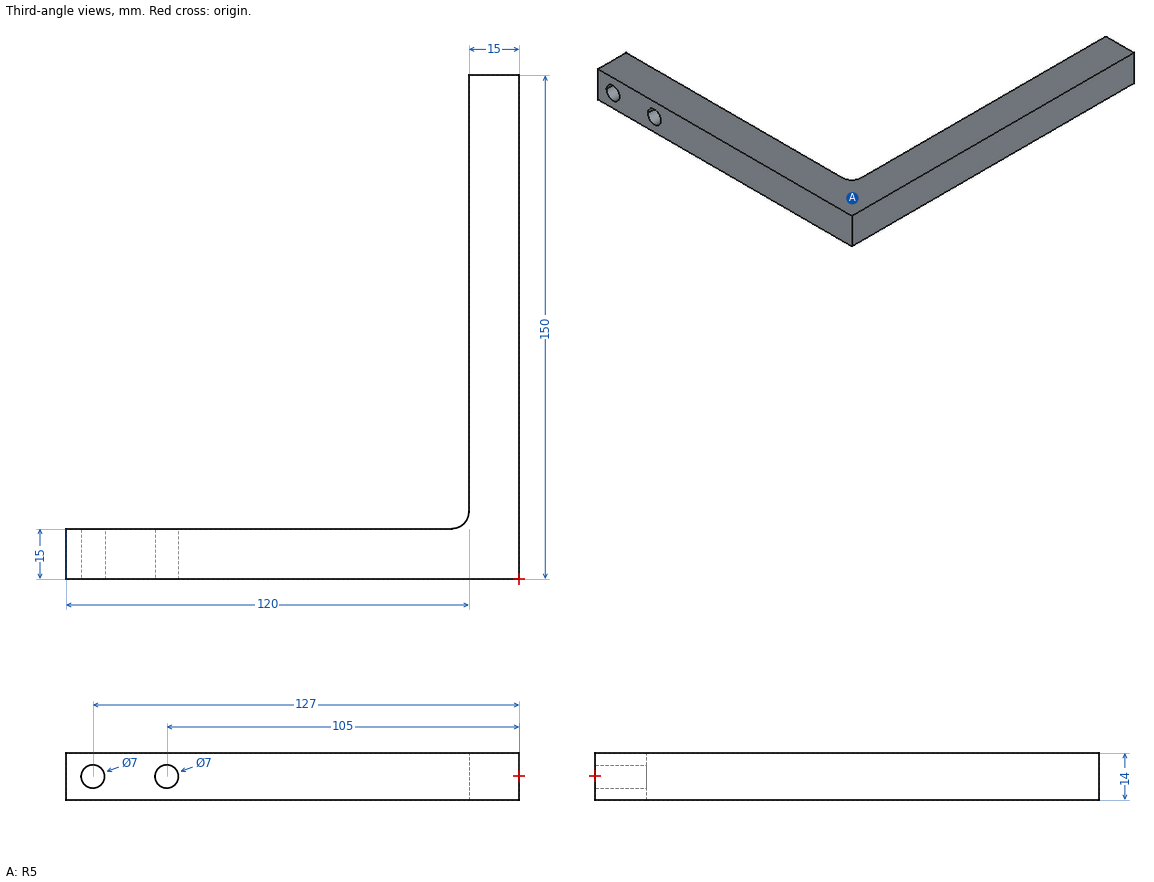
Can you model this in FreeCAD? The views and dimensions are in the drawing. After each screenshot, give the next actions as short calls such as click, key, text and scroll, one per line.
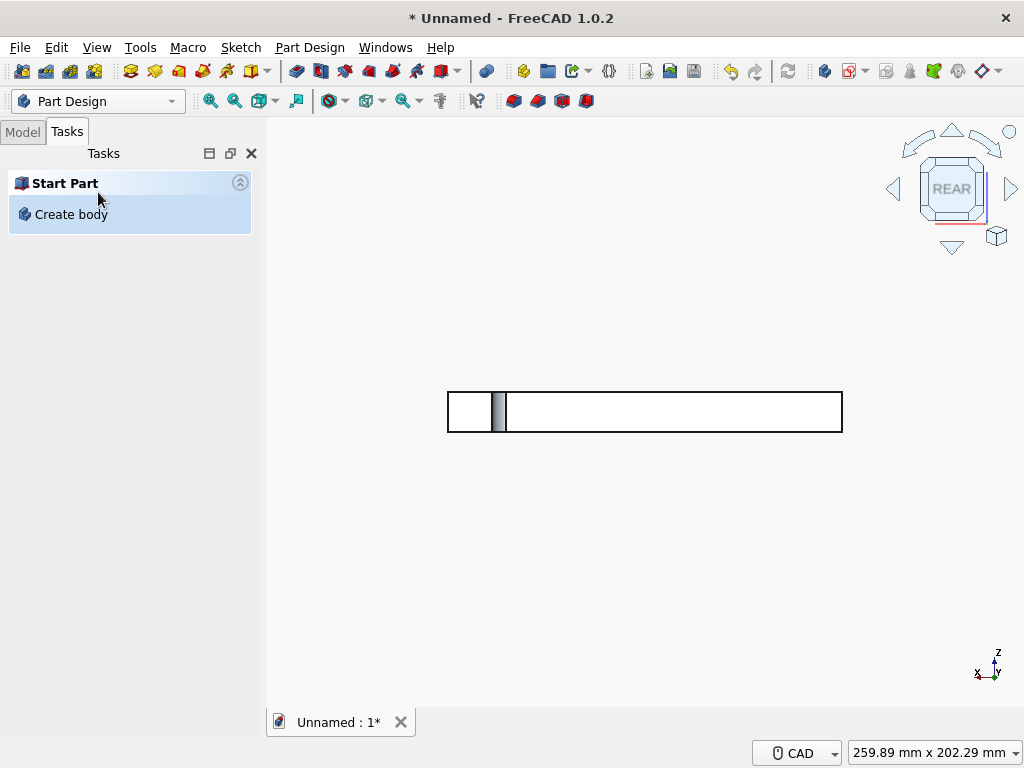
click(530, 411)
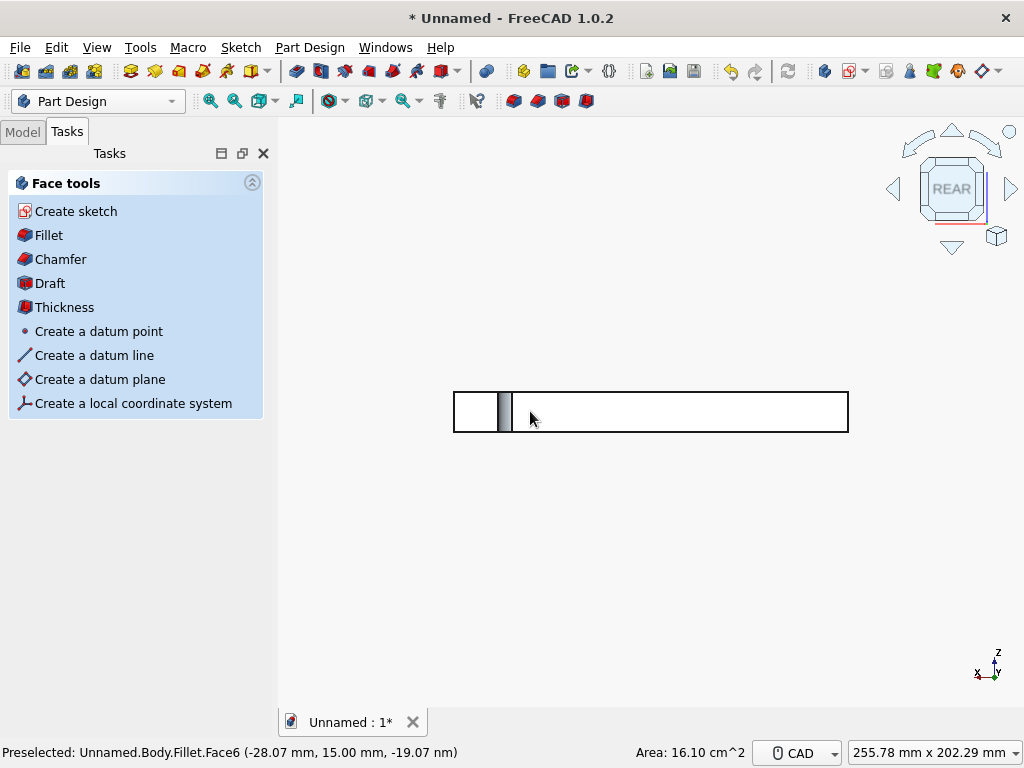
click(850, 72)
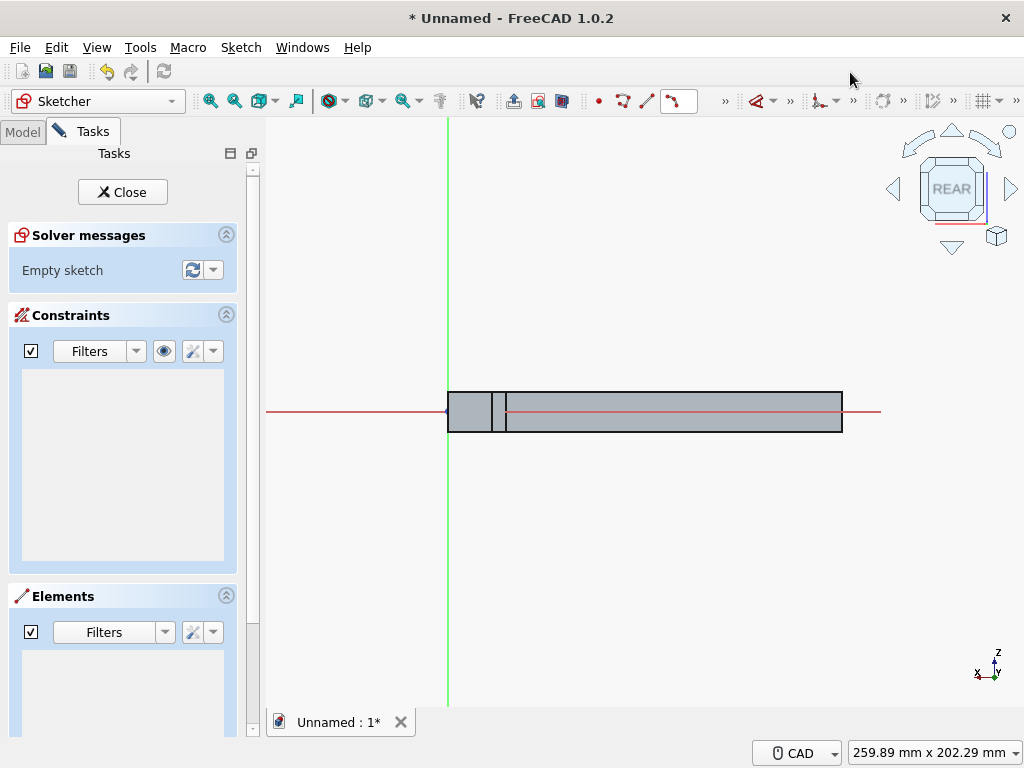
scroll(831, 412, up, 15)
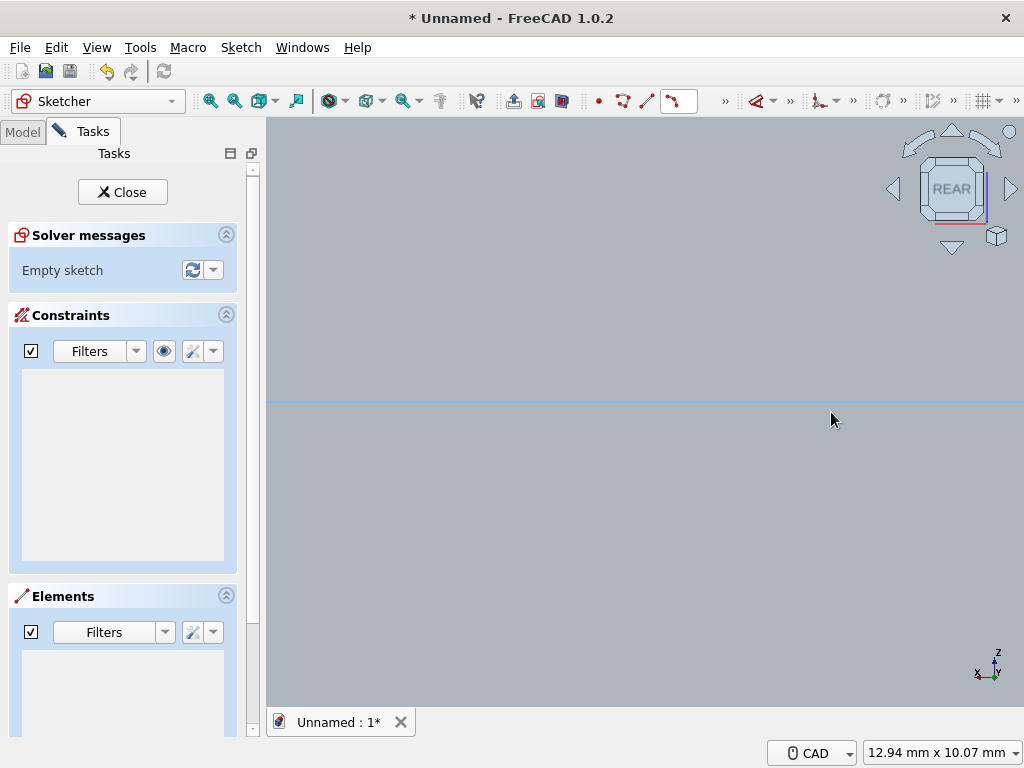
key(g)
key(c)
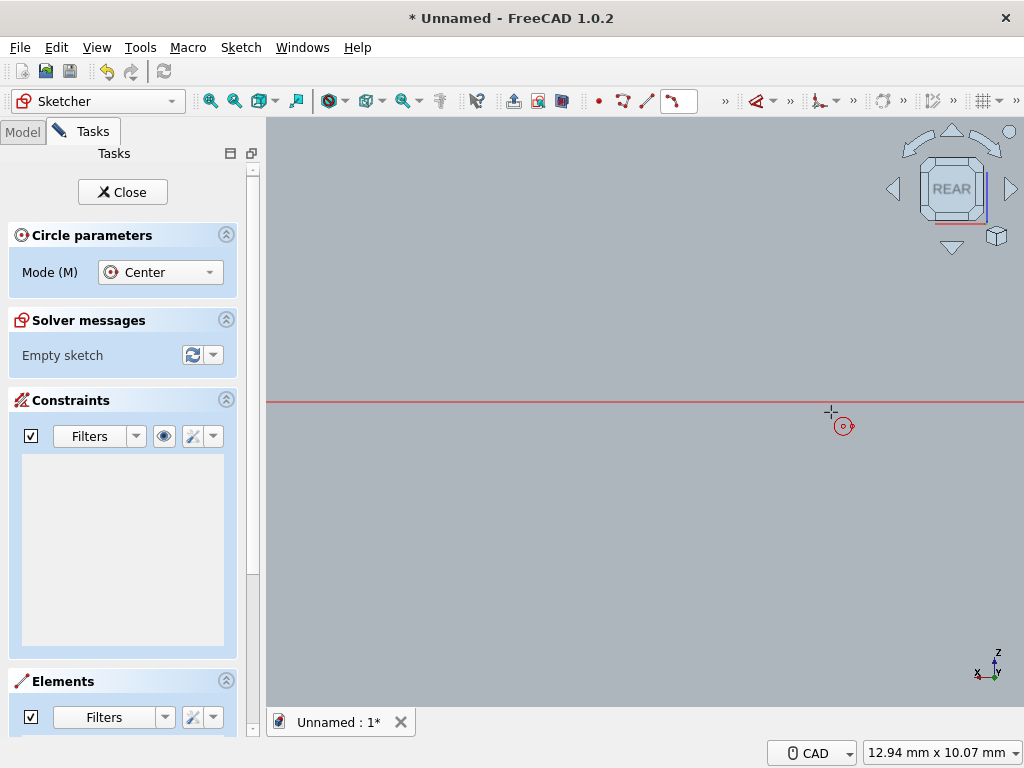
click(566, 402)
click(711, 257)
key(Escape)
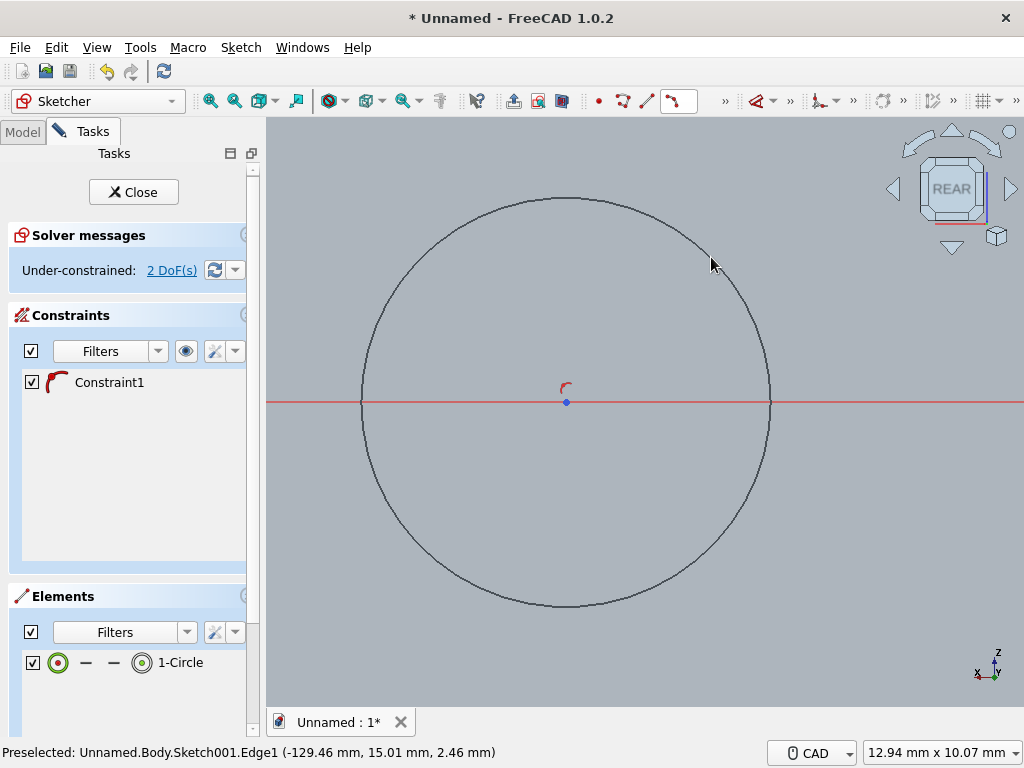
click(756, 102)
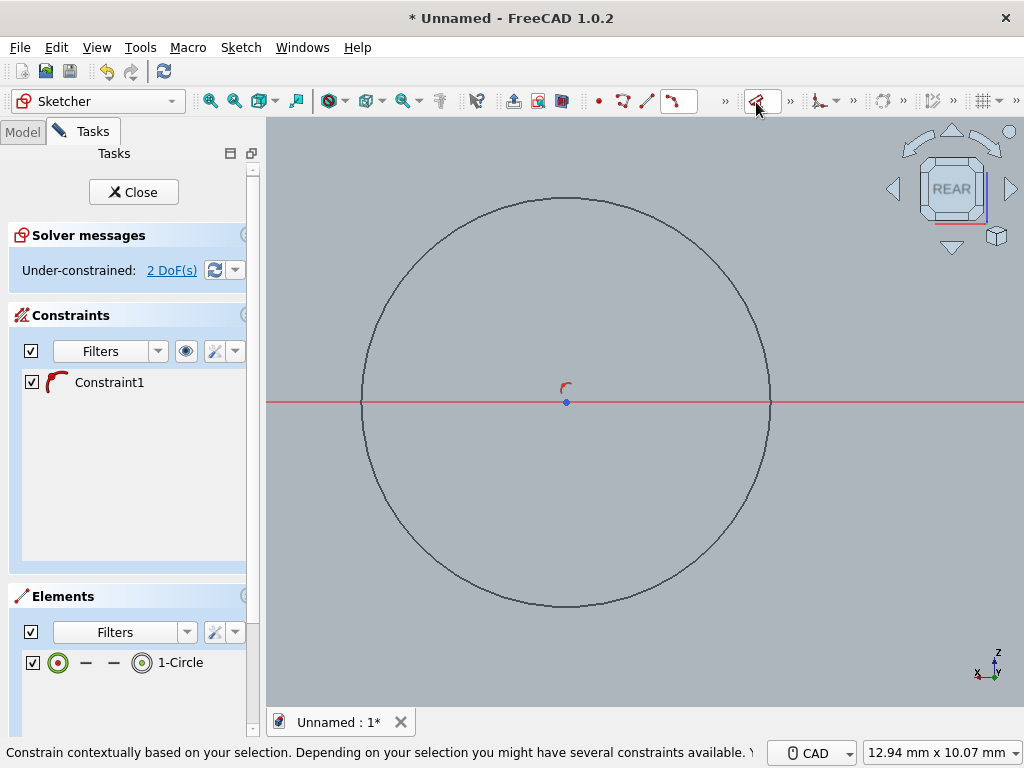
click(710, 257)
click(733, 234)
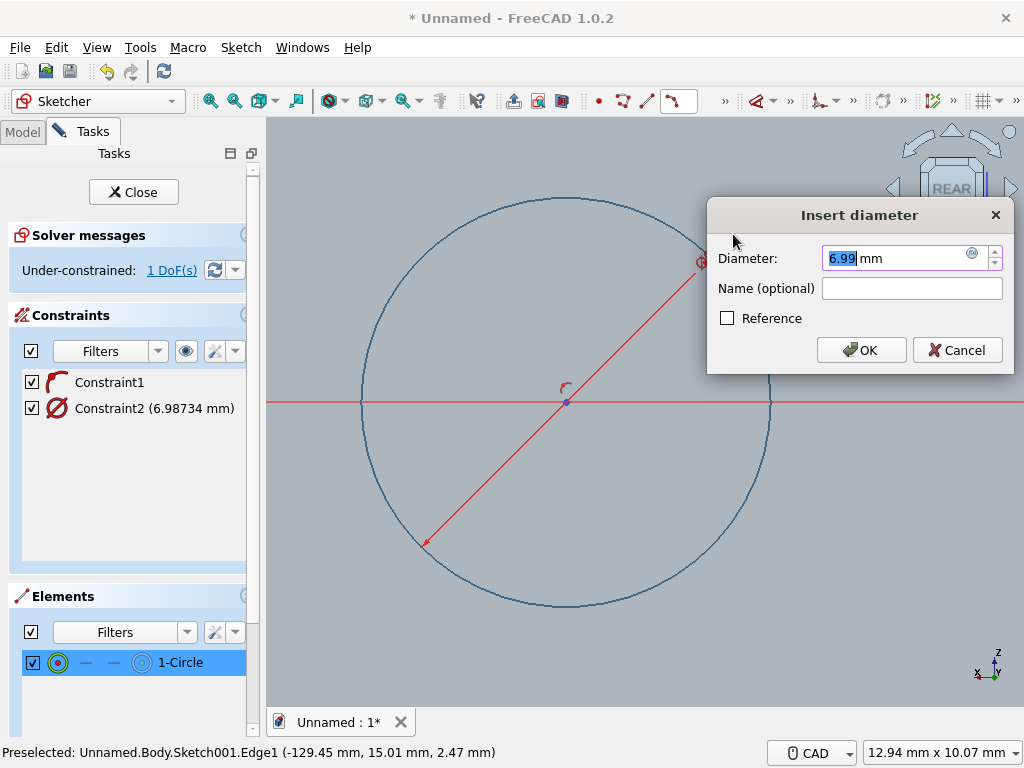
text(7)
key(Return)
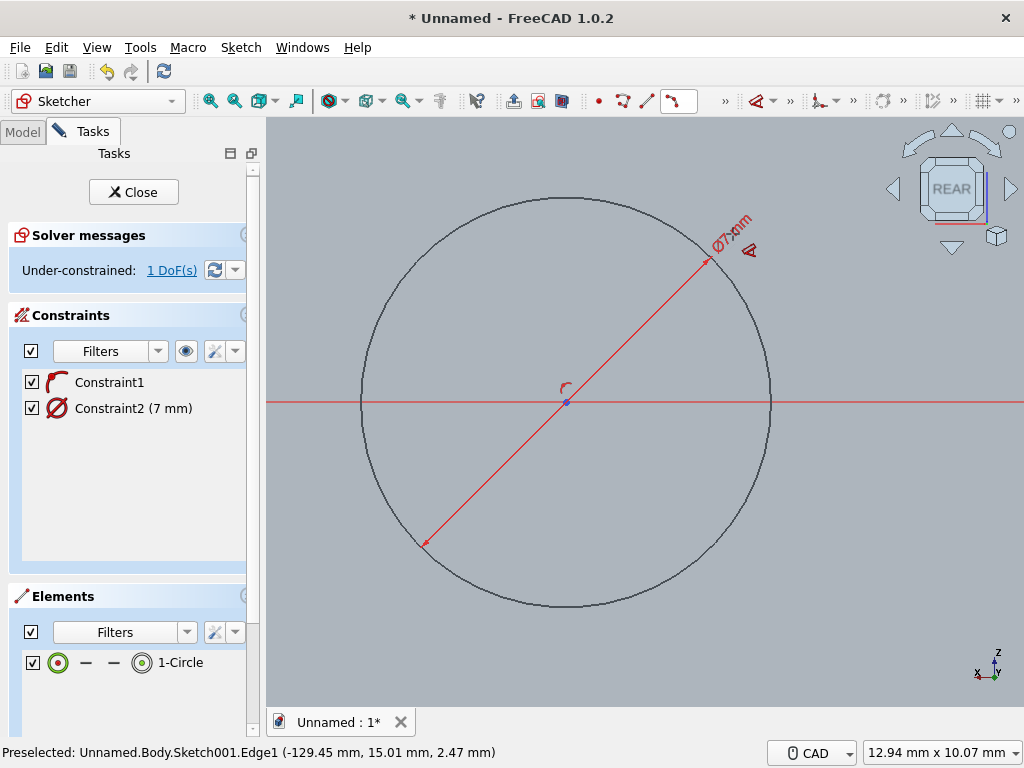
click(566, 402)
click(430, 436)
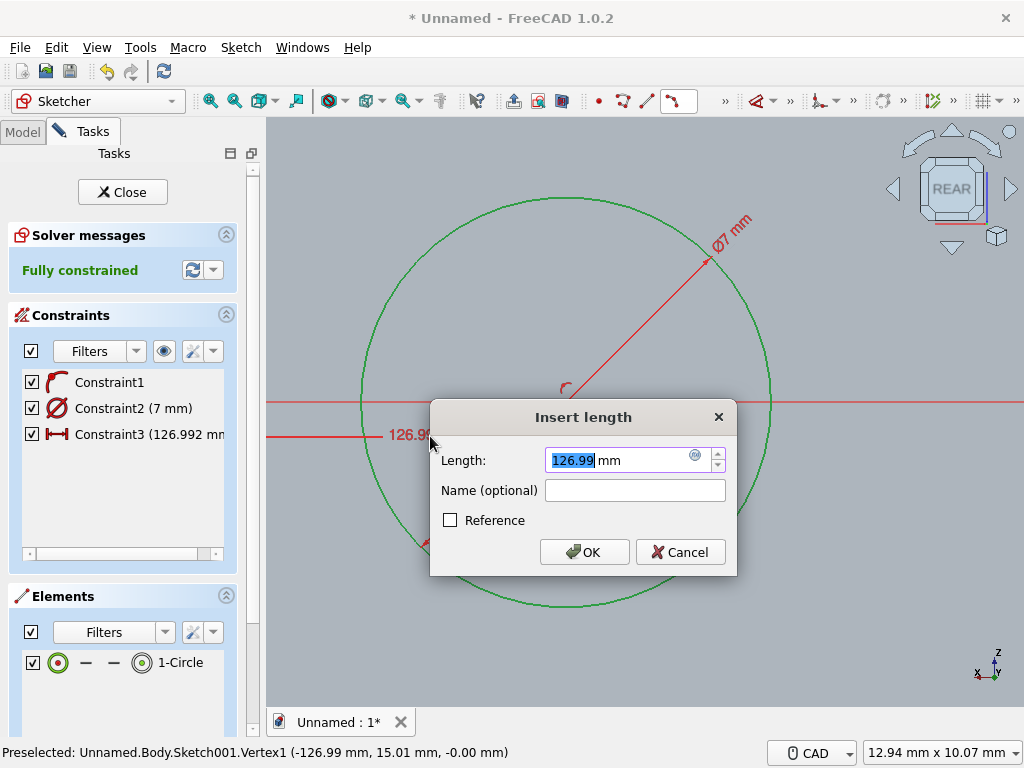
text(127)
key(Return)
key(Escape)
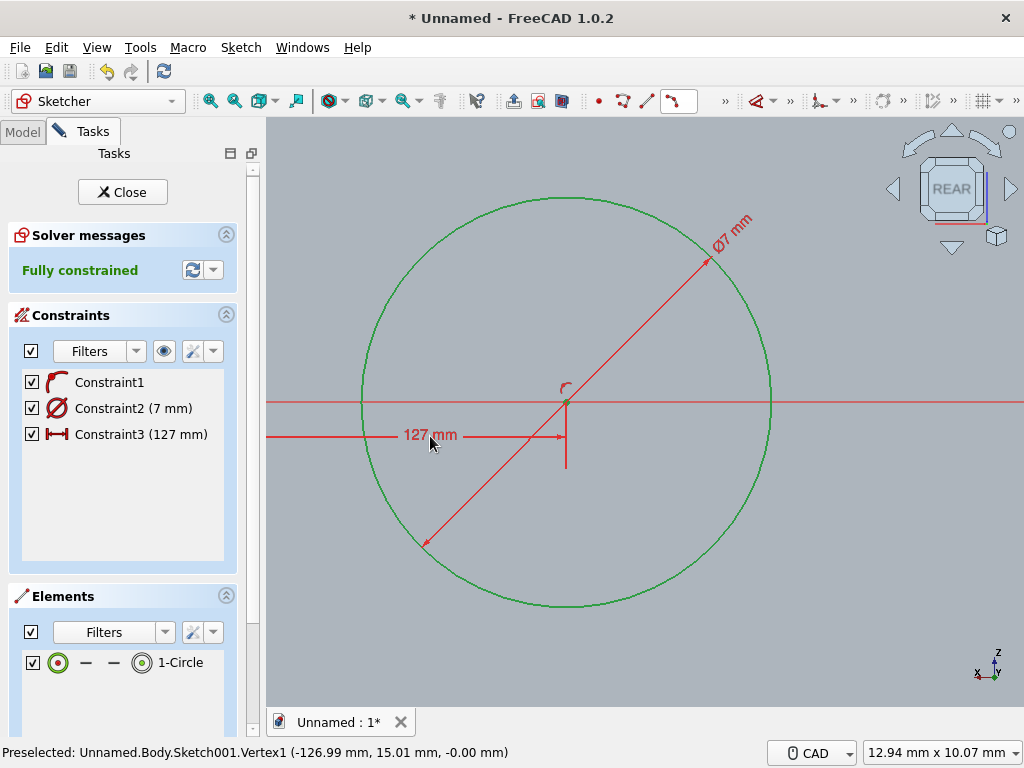
click(123, 192)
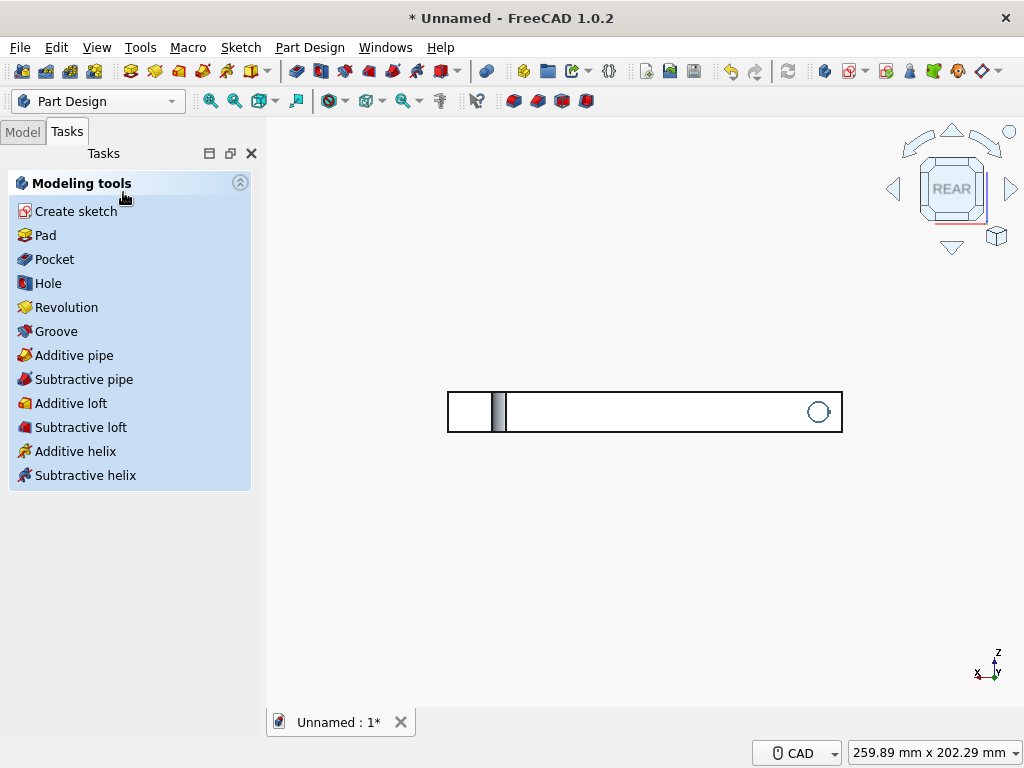
click(298, 72)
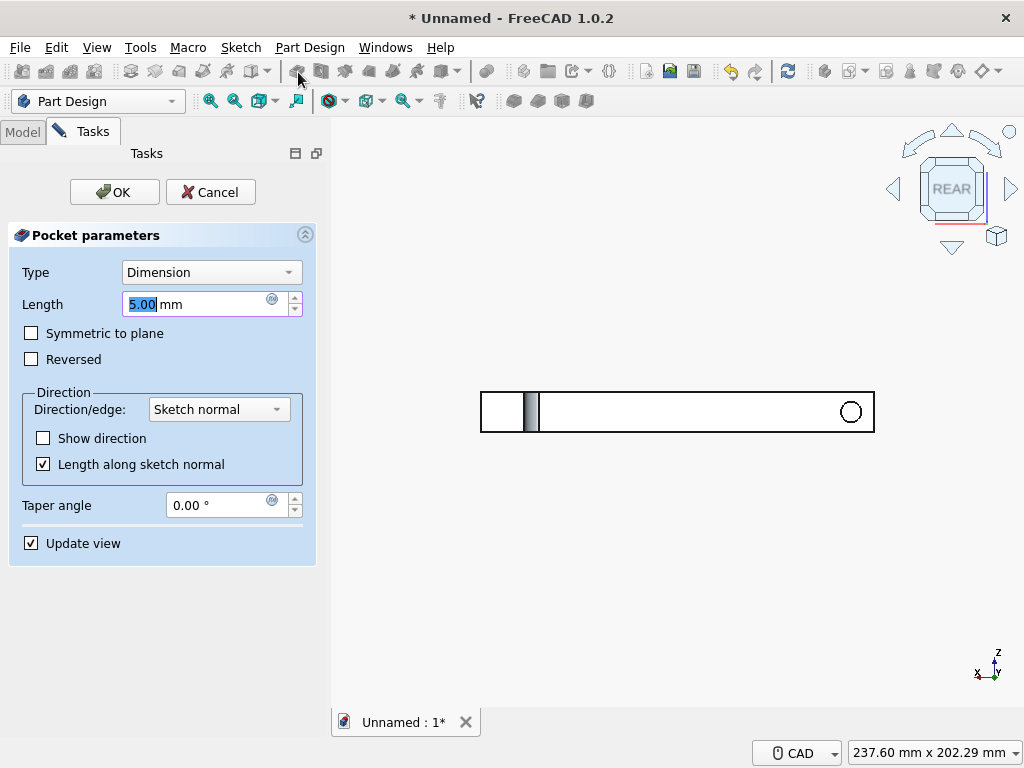
click(212, 272)